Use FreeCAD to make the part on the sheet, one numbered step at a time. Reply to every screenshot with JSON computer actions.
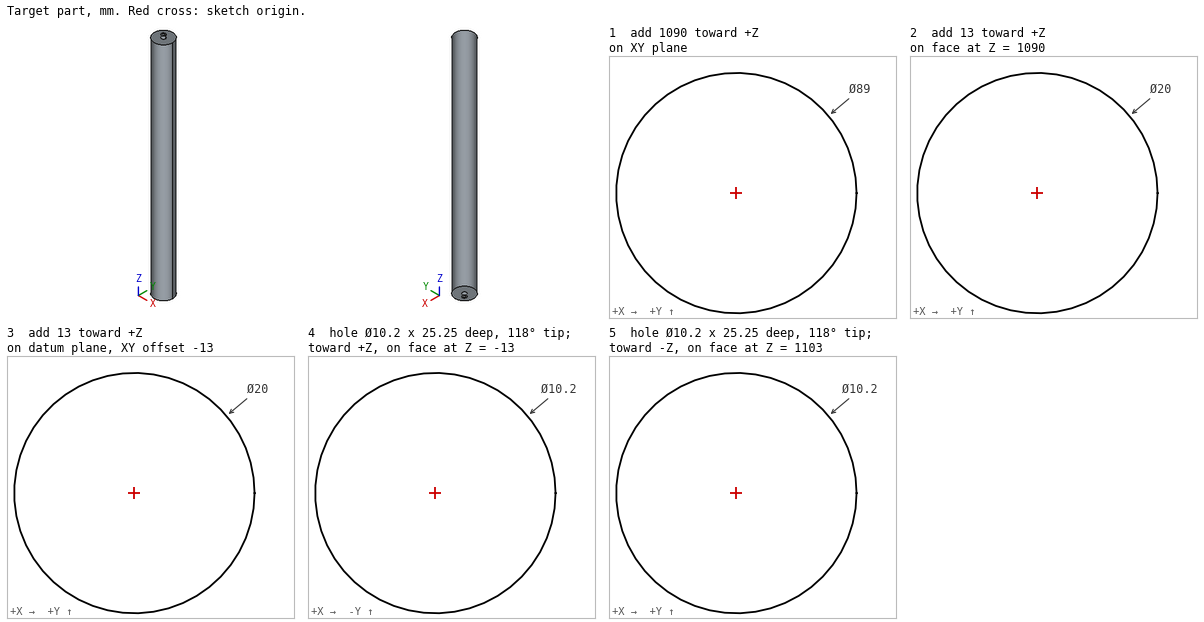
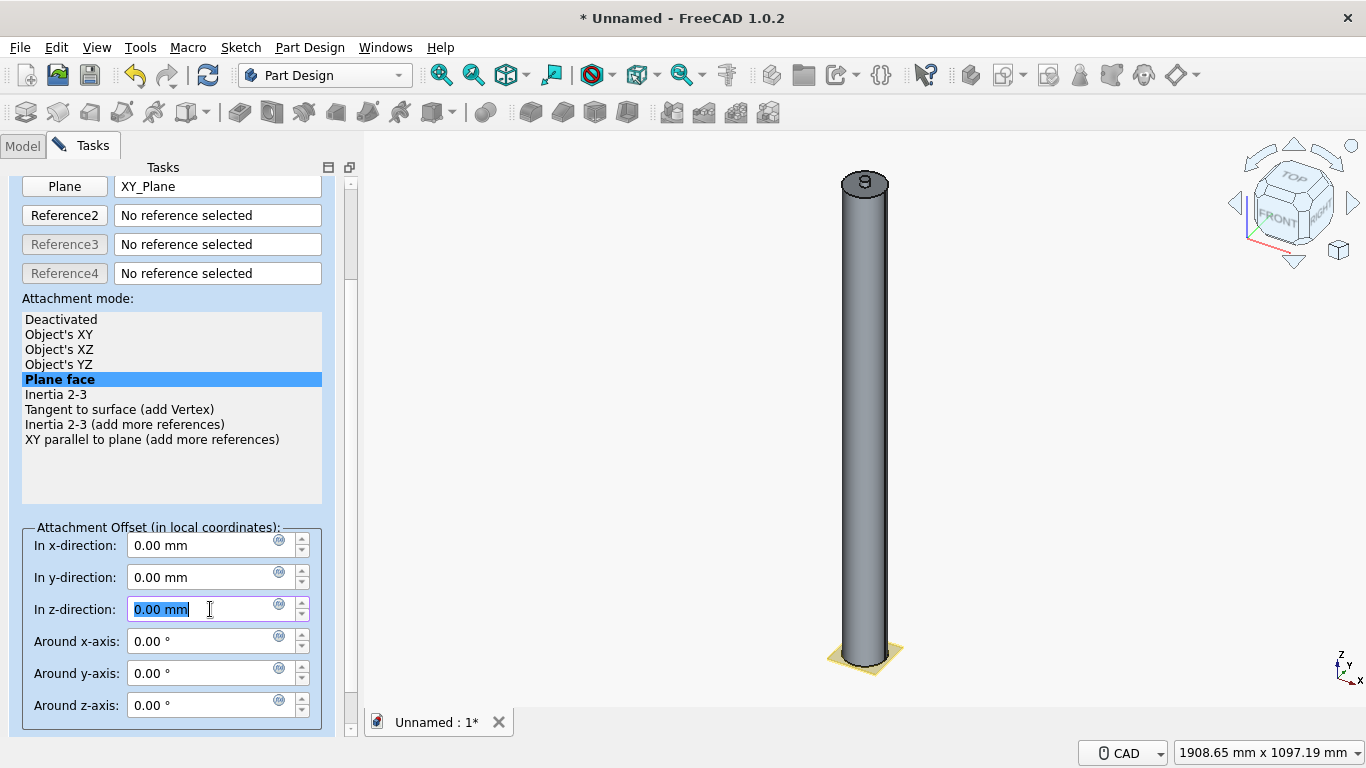
{"action": "type", "text": "-13"}
{"action": "key", "text": "Tab"}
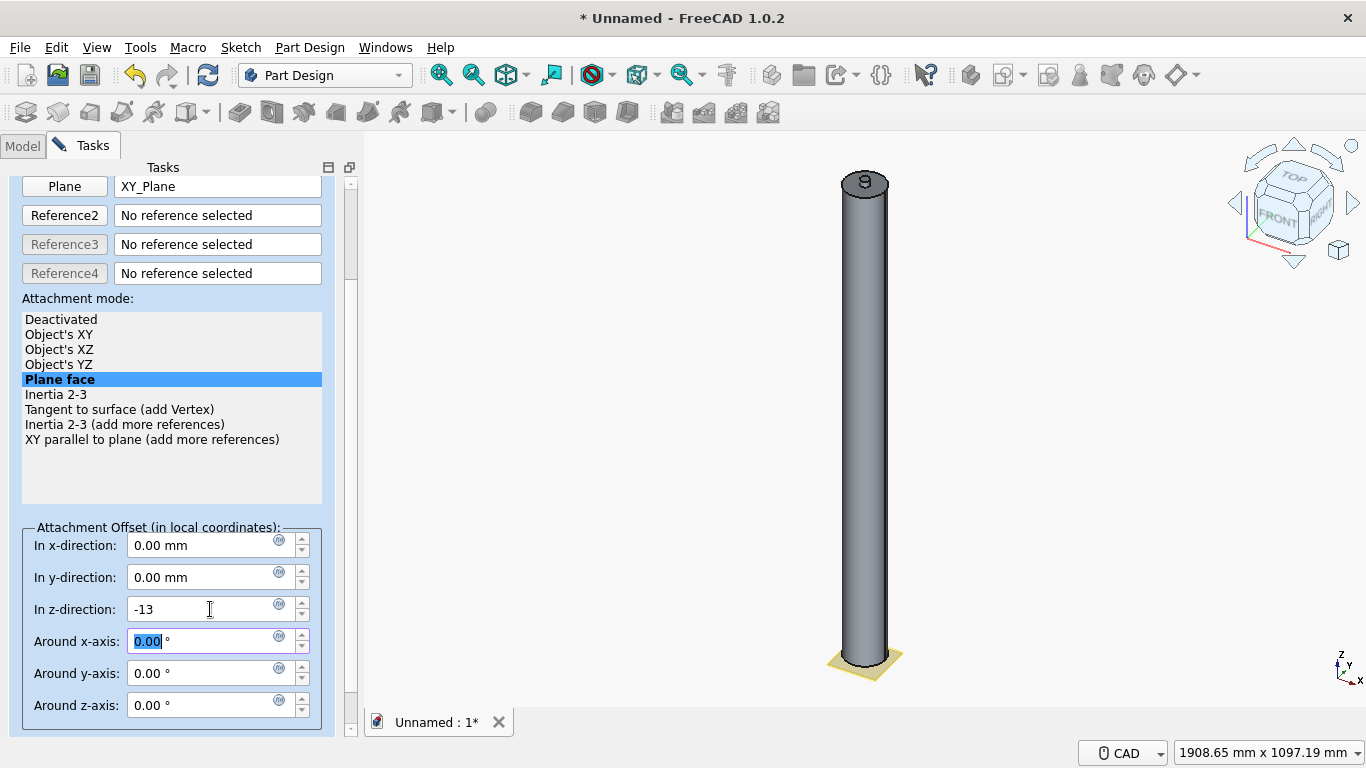
{"action": "scroll", "coordinate": [351, 456], "scroll_direction": "up", "scroll_amount": 3}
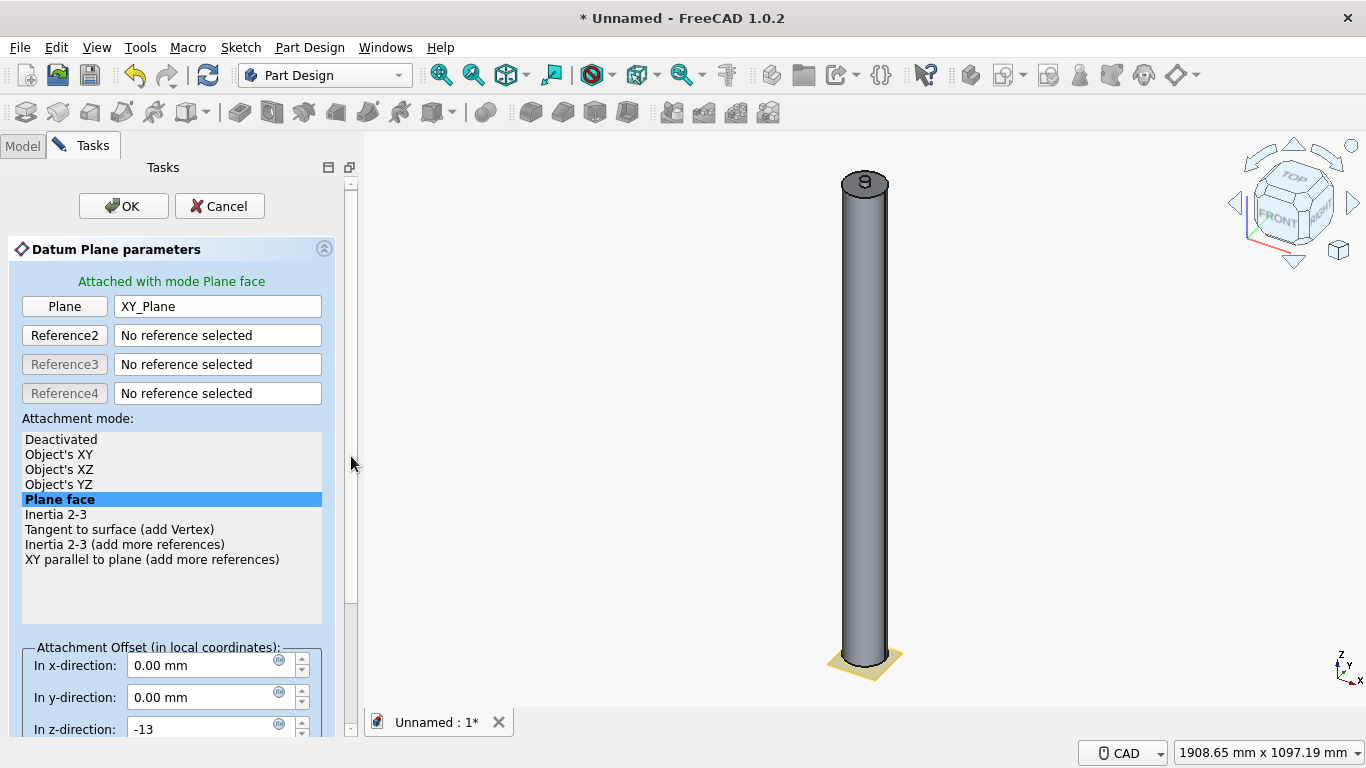
{"action": "left_click", "coordinate": [124, 206]}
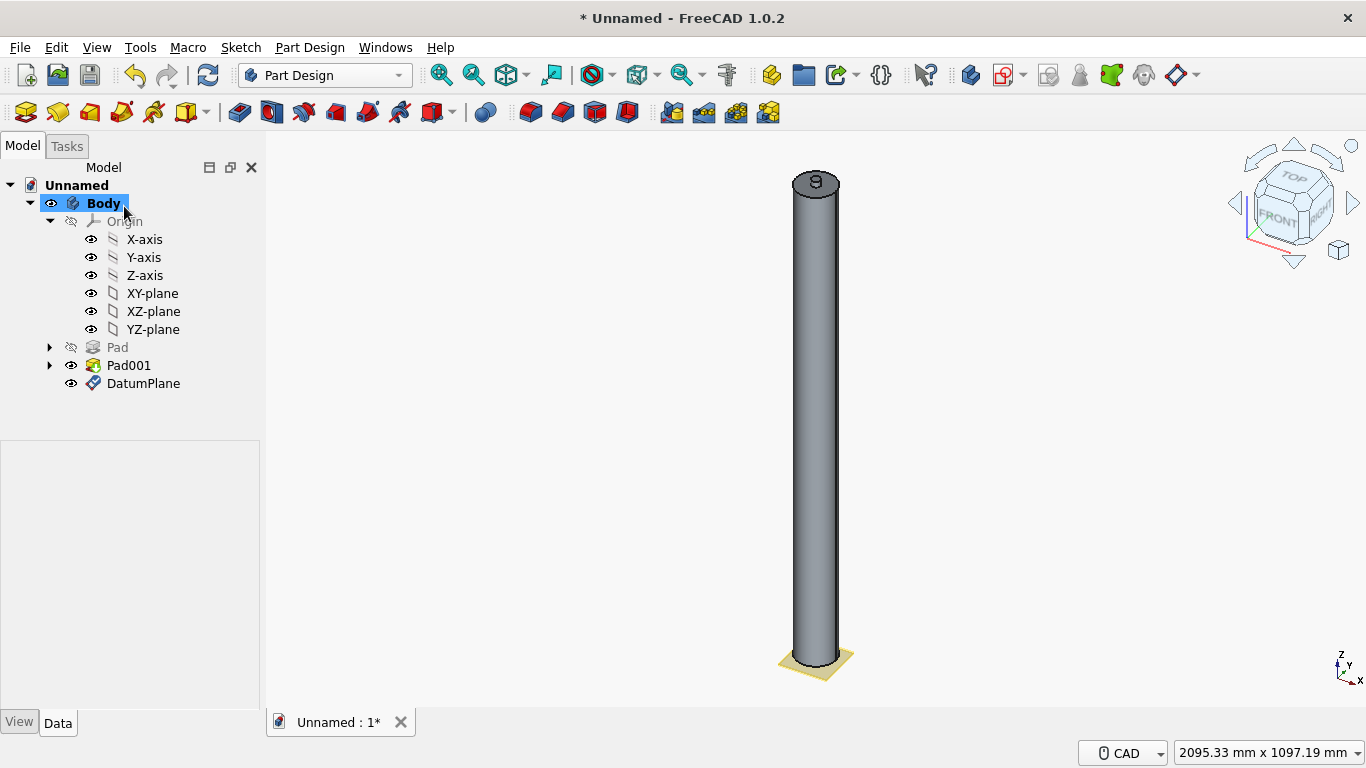
{"action": "left_click", "coordinate": [116, 383]}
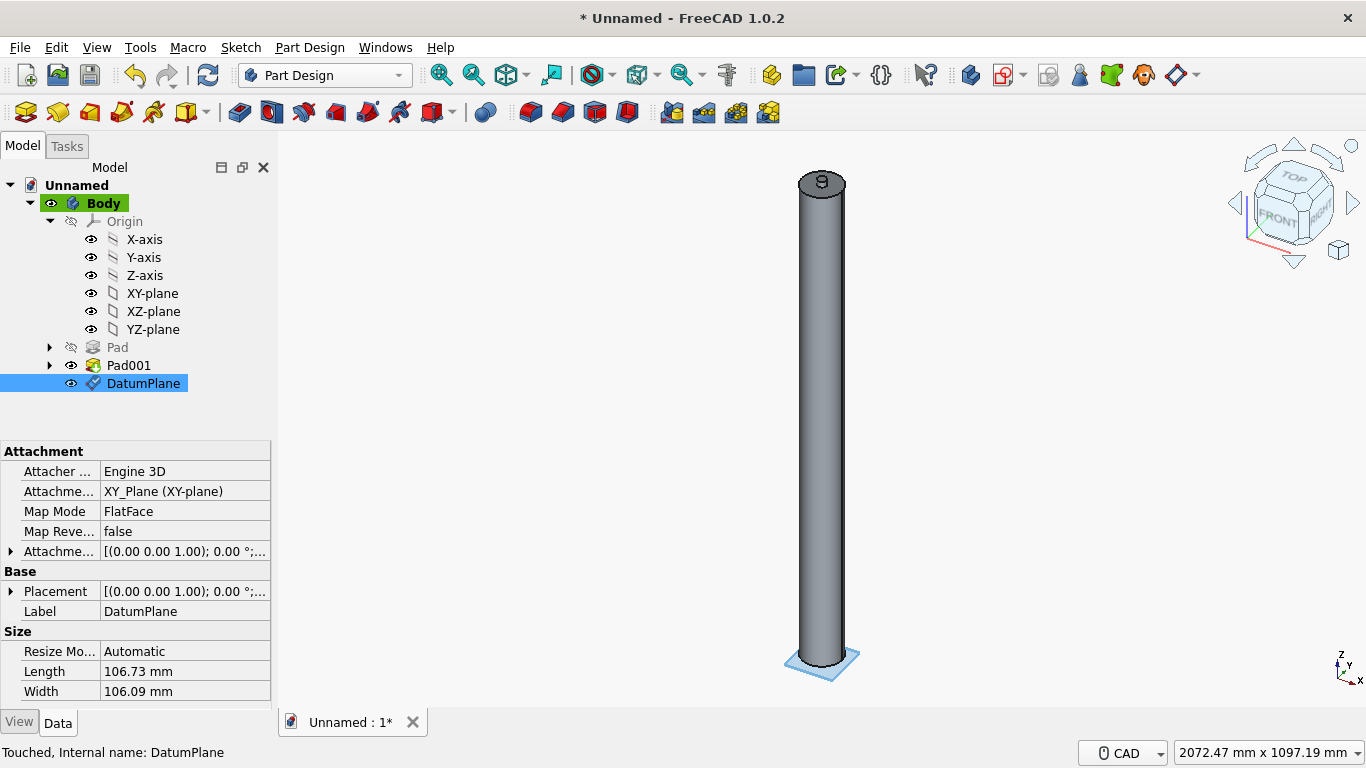
{"action": "left_click", "coordinate": [1004, 76]}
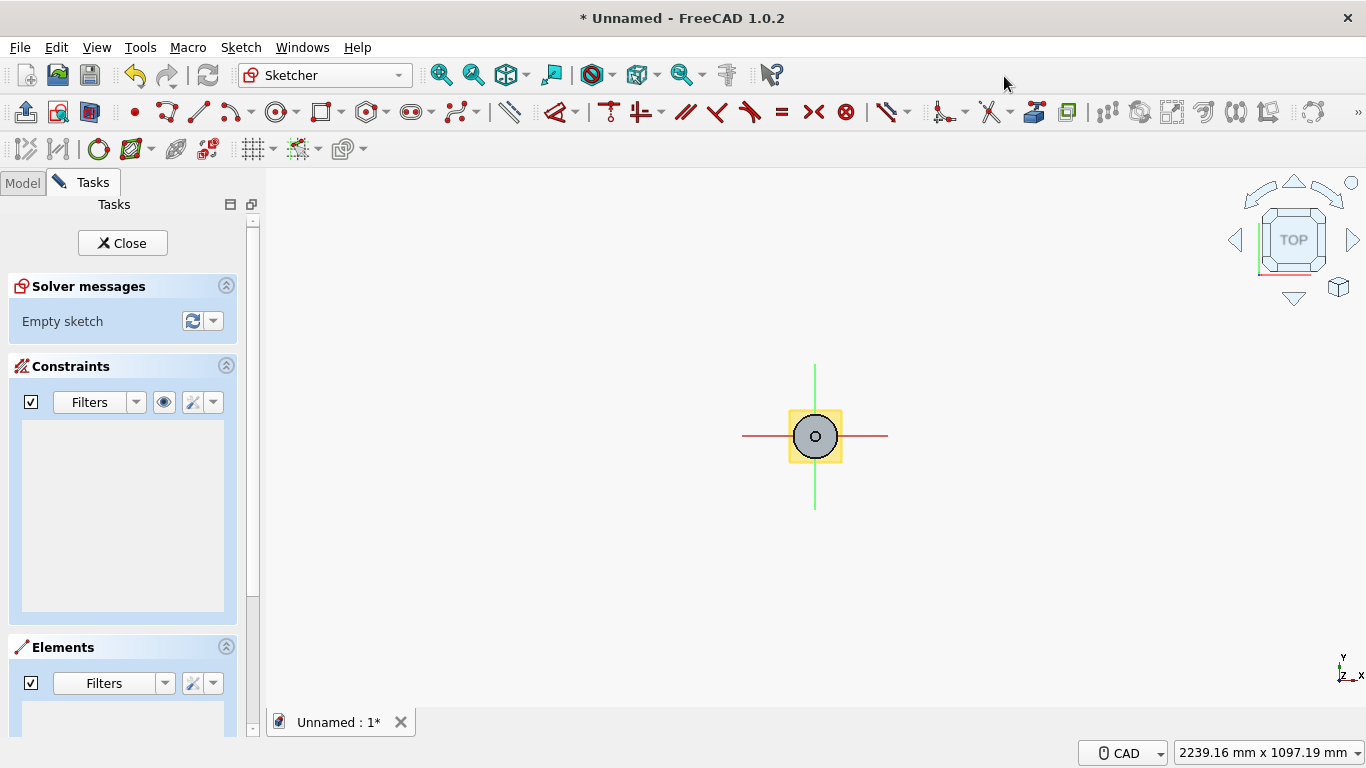
{"action": "key", "text": "q s"}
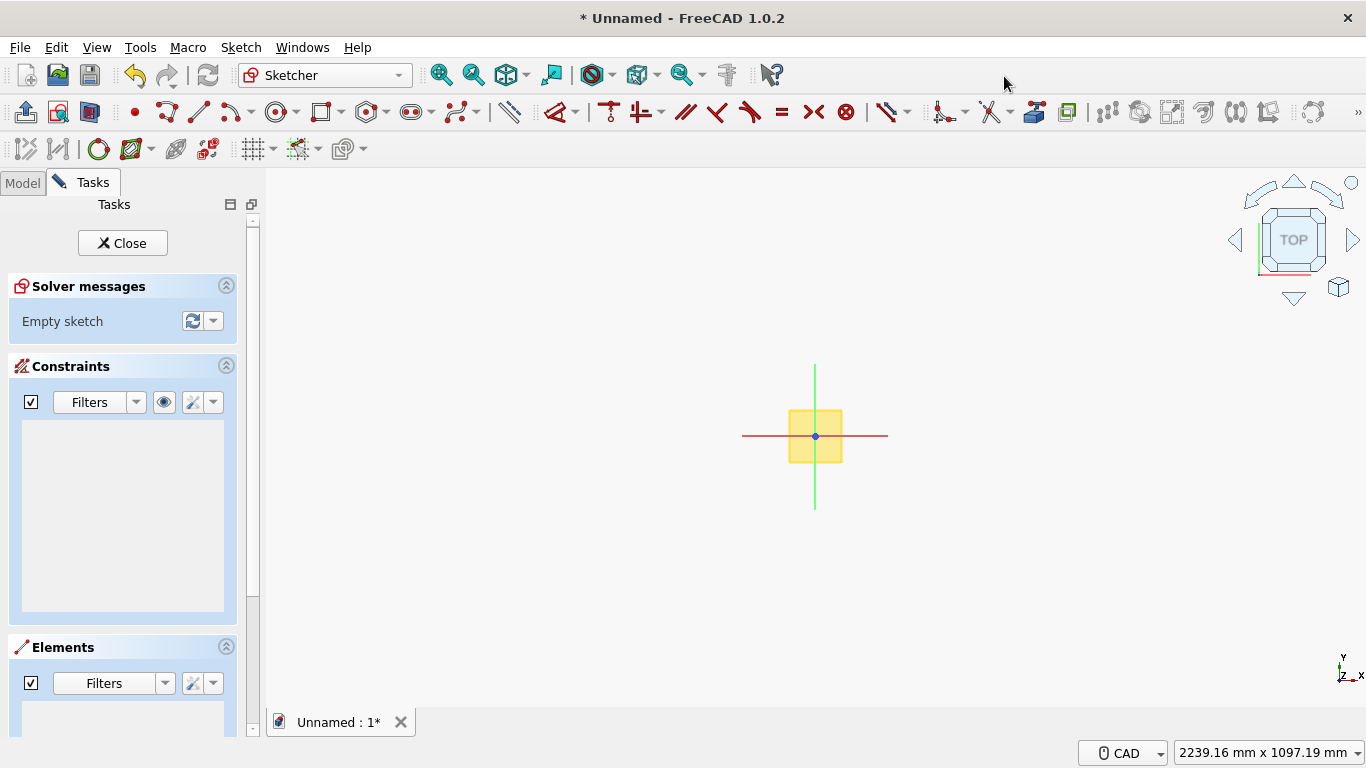
{"action": "scroll", "coordinate": [819, 436], "scroll_direction": "up", "scroll_amount": 15}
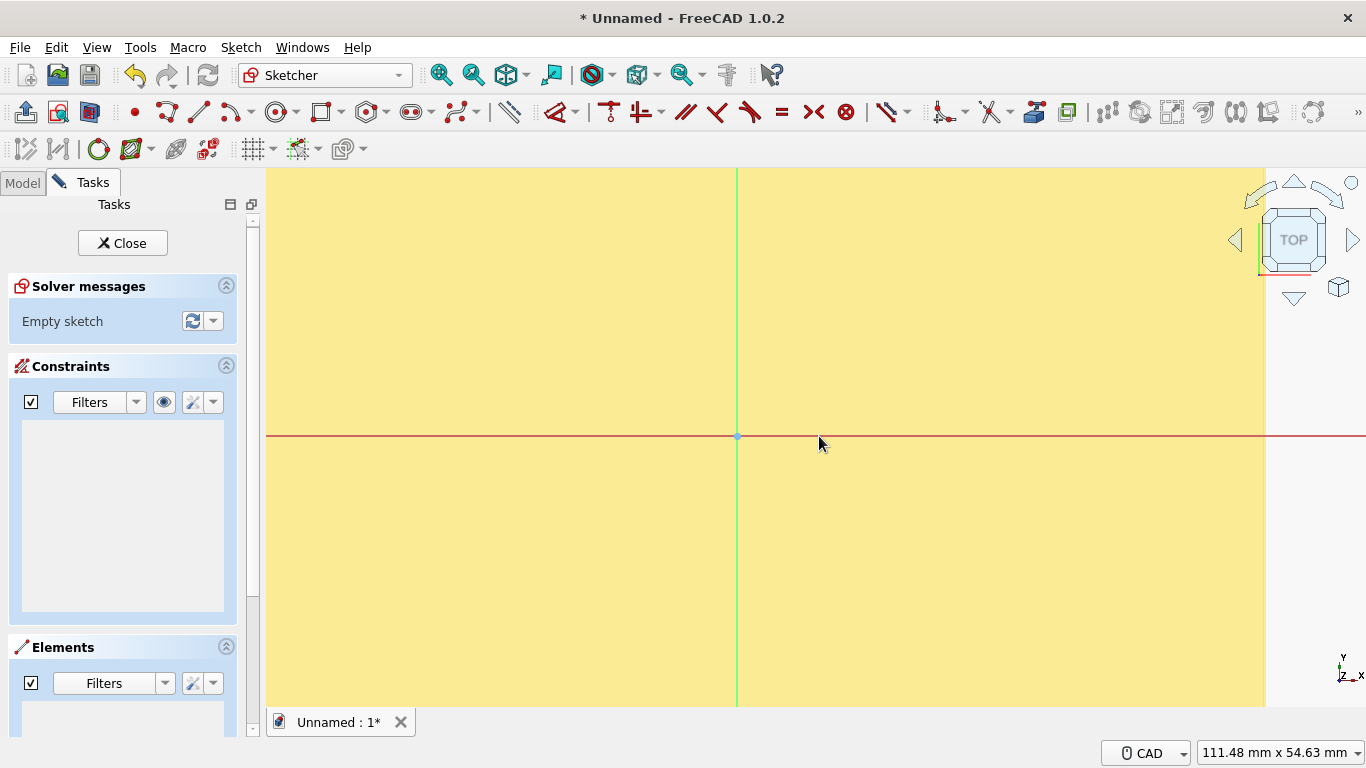
{"action": "scroll", "coordinate": [725, 435], "scroll_direction": "up", "scroll_amount": 3}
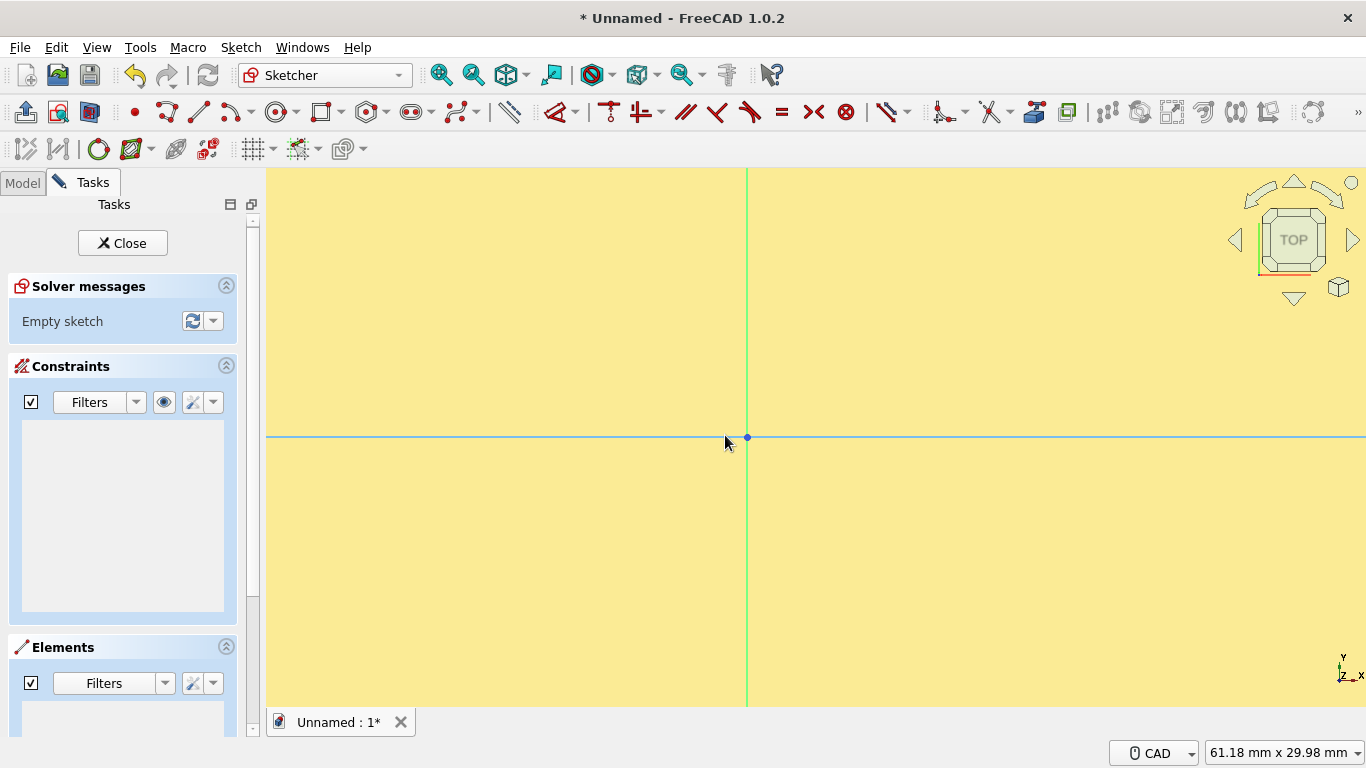
{"action": "left_click", "coordinate": [276, 112]}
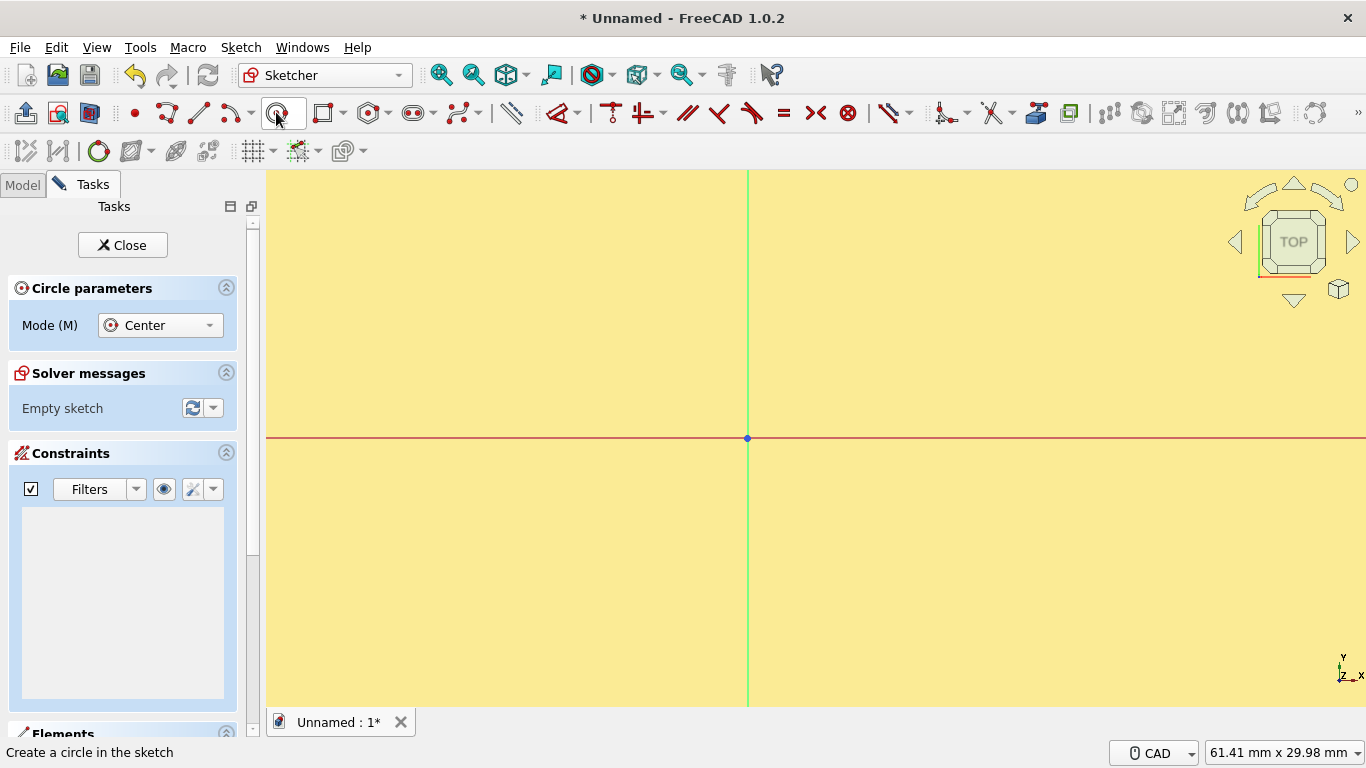
{"action": "left_click", "coordinate": [748, 438]}
{"action": "mouse_move", "coordinate": [874, 311]}